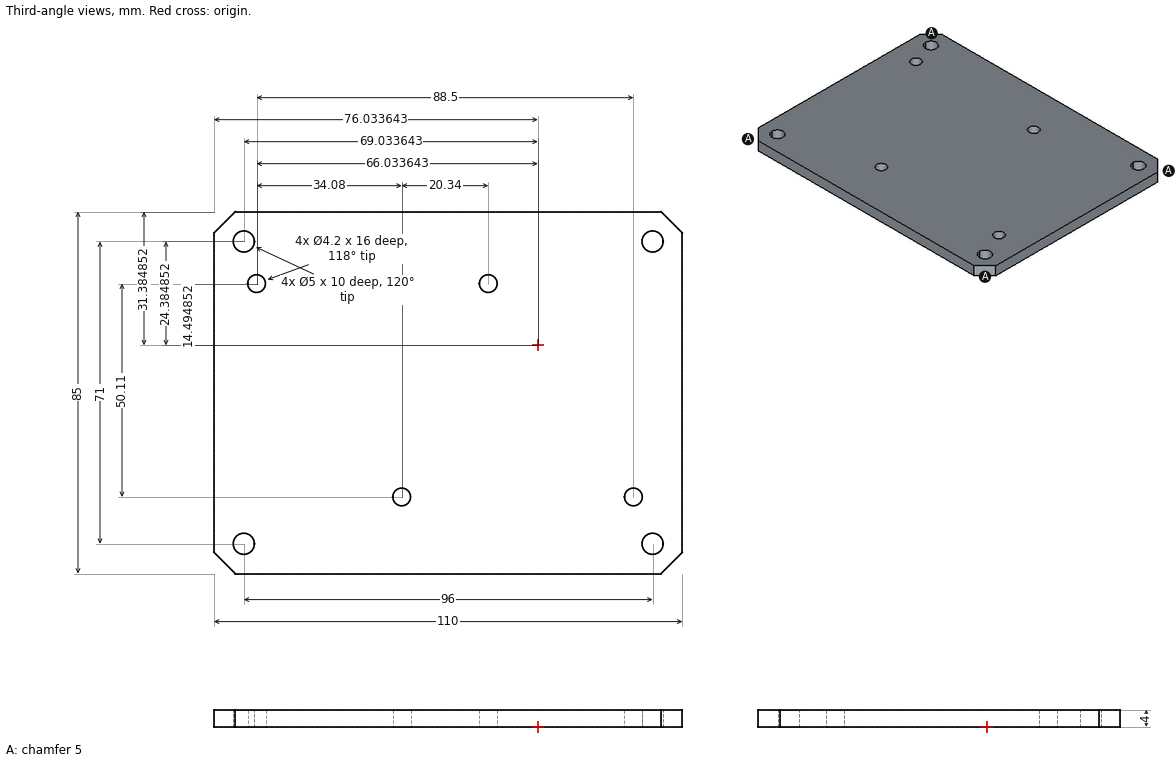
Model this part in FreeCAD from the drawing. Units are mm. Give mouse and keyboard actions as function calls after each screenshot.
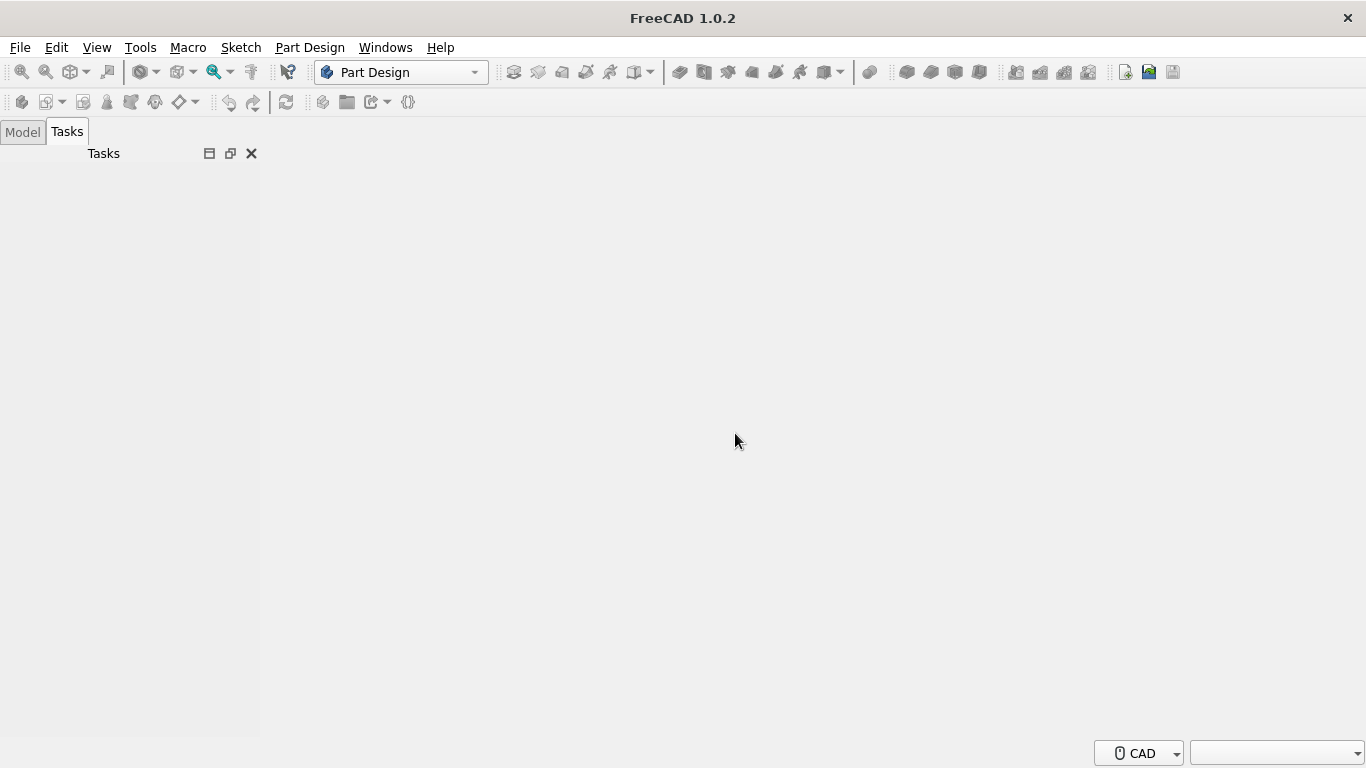
click(1126, 72)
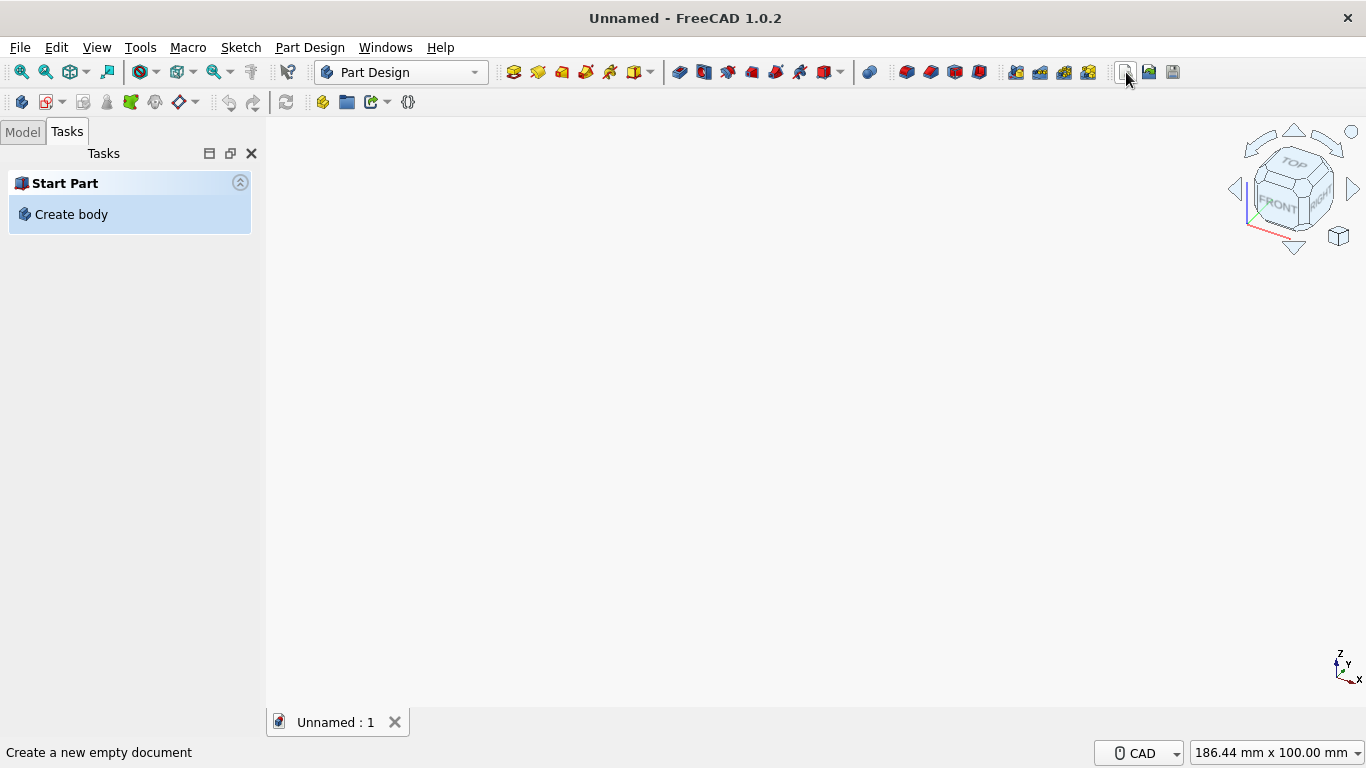
click(46, 102)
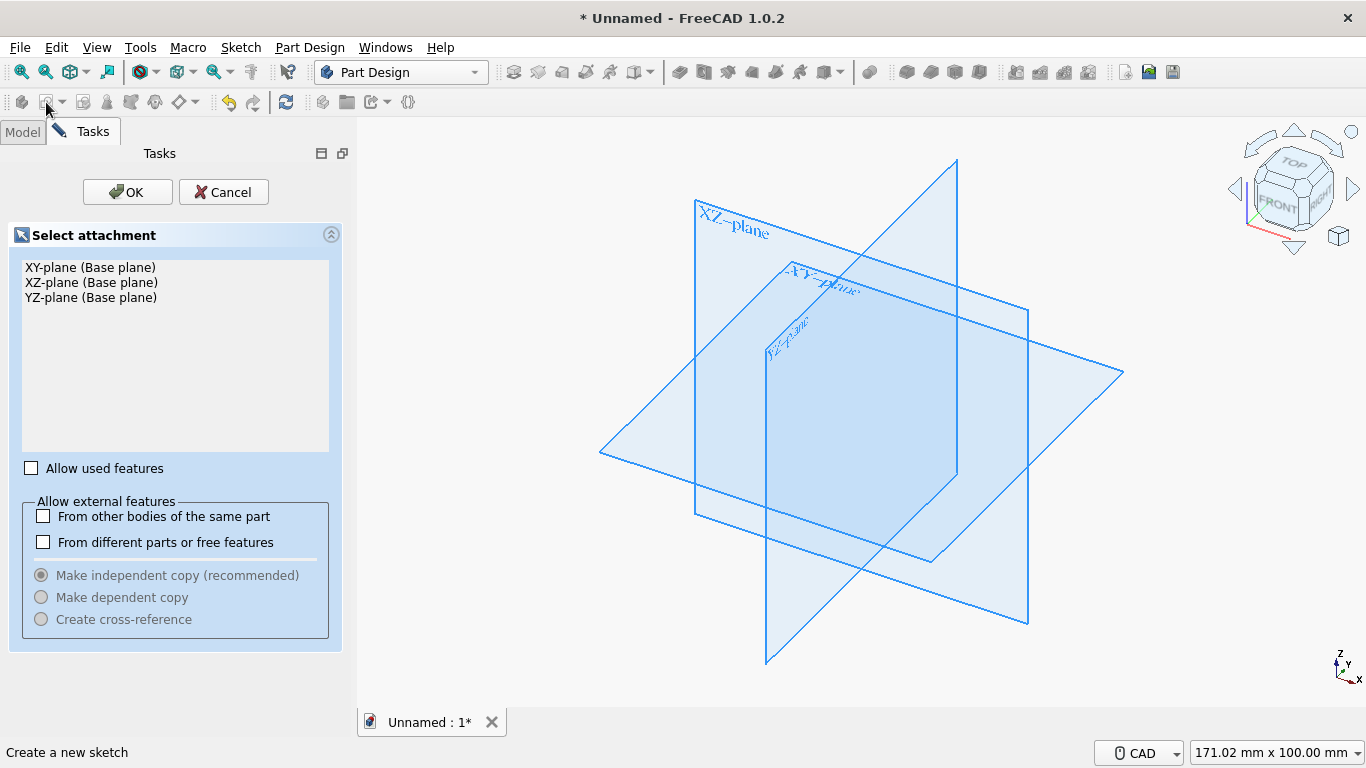
click(82, 268)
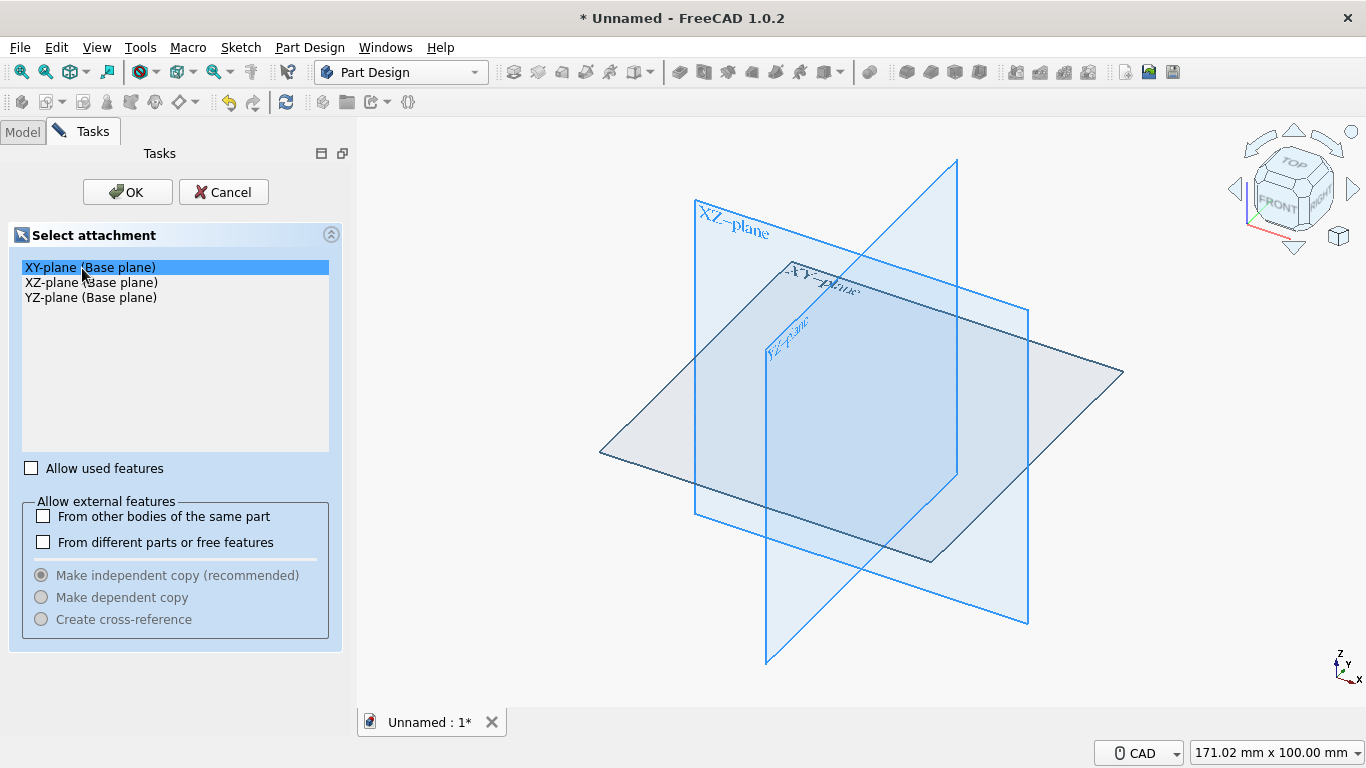
click(128, 192)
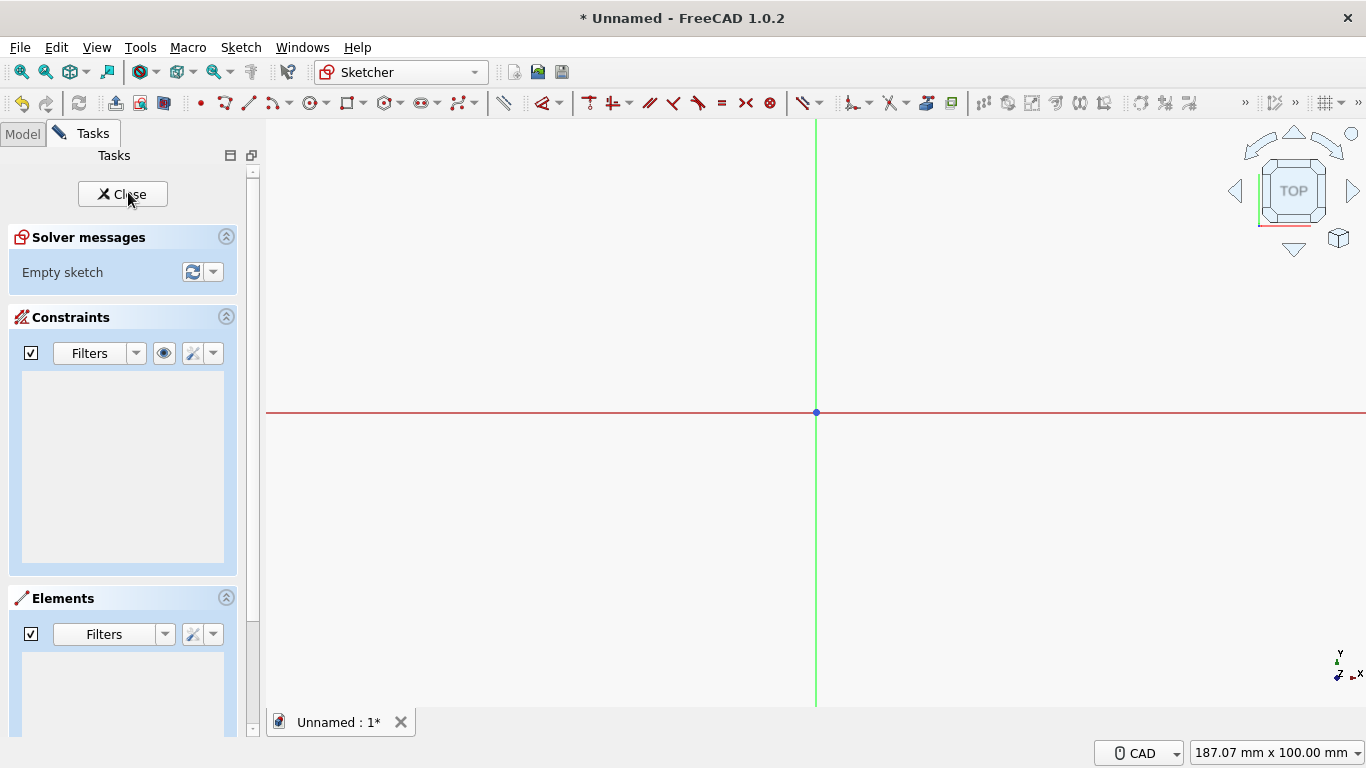
scroll(997, 147, down, 1)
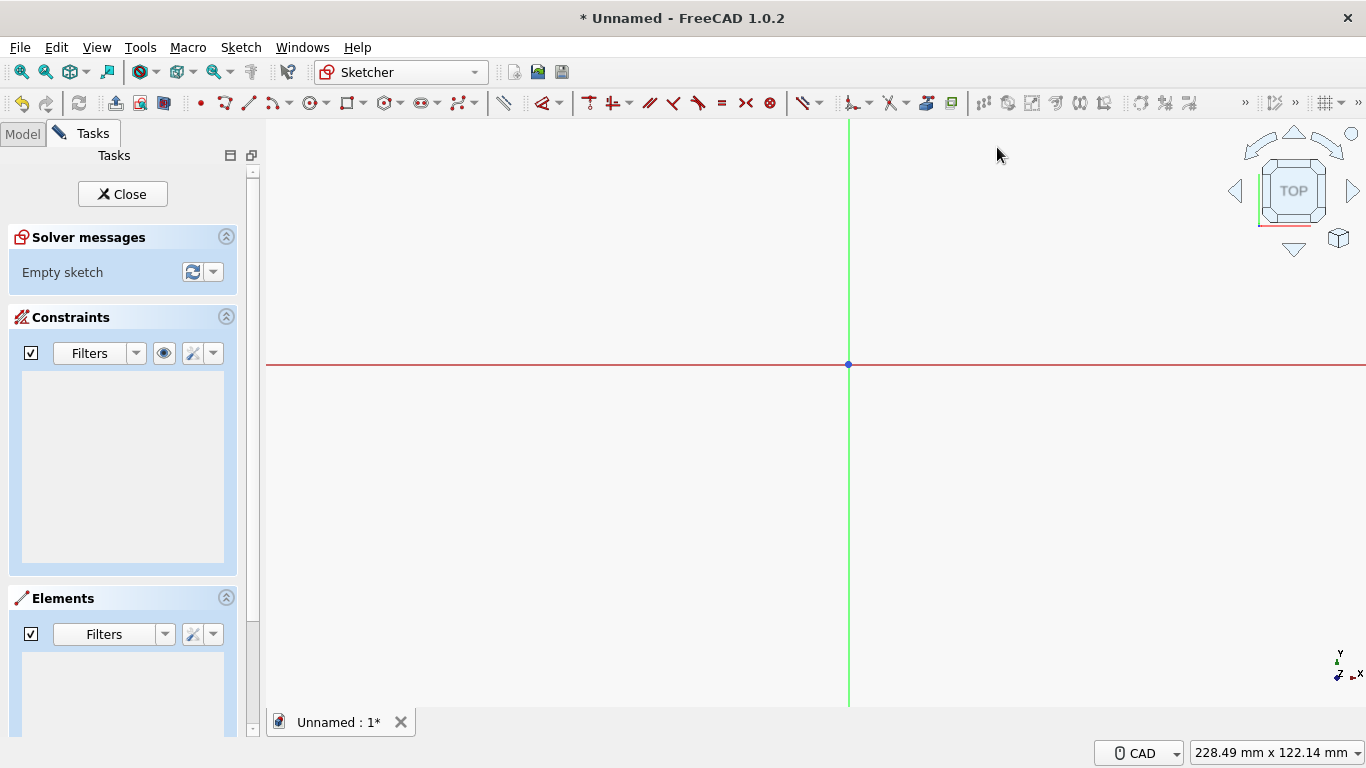
click(348, 104)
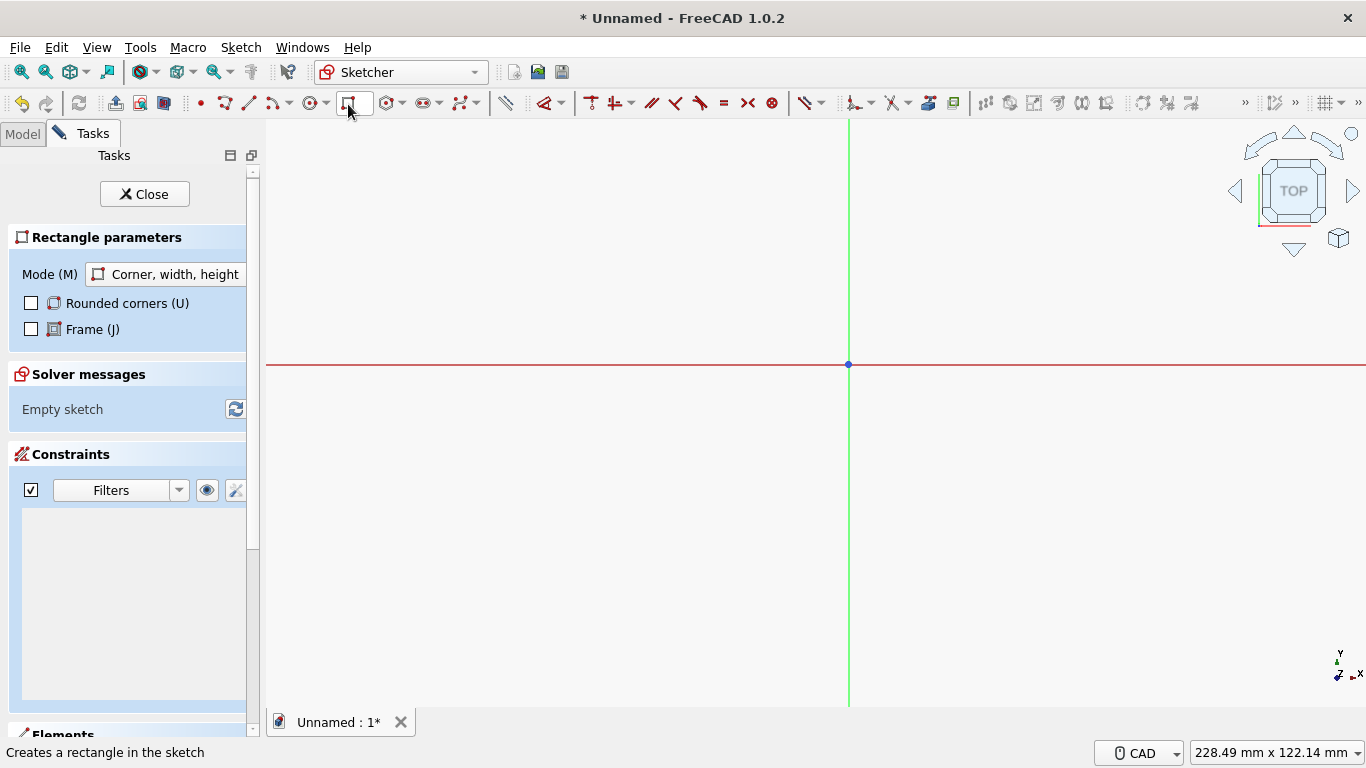
click(483, 214)
click(1012, 623)
key(Escape)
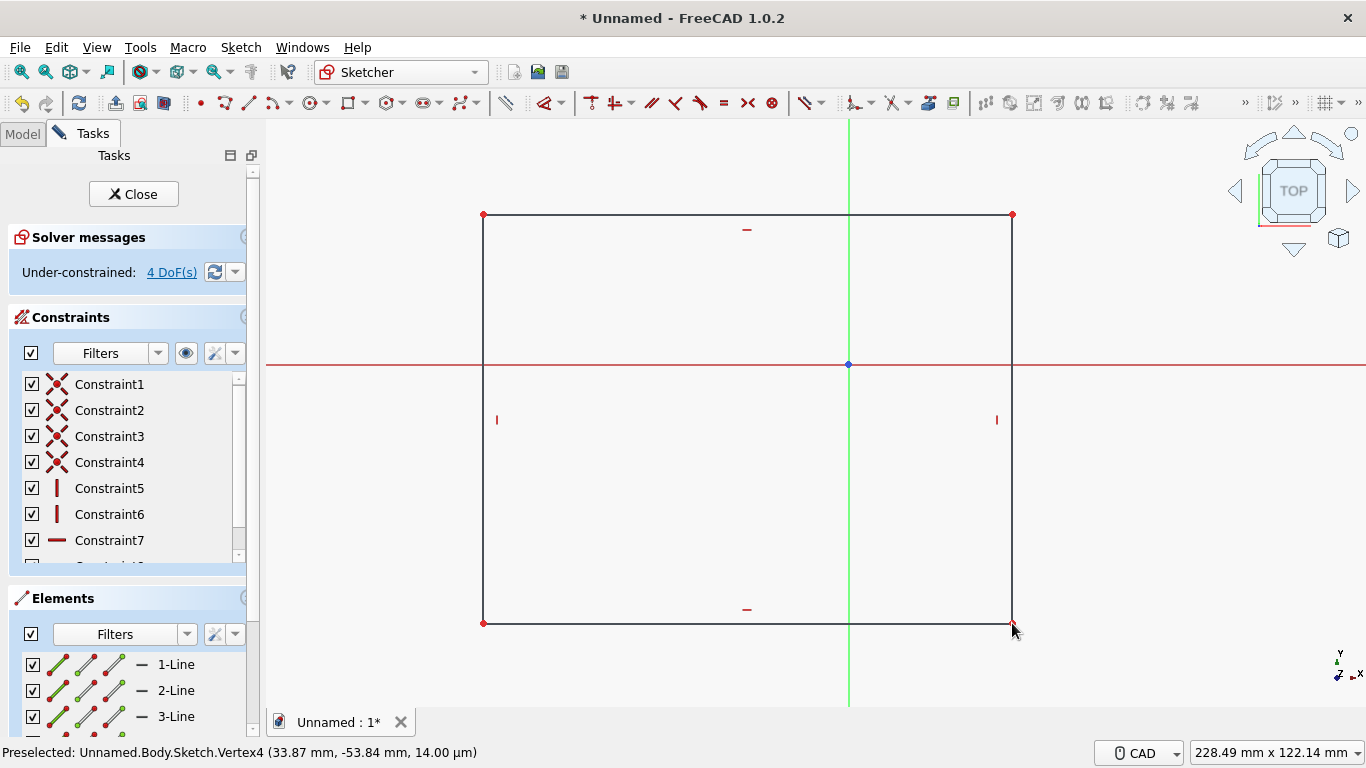
click(544, 104)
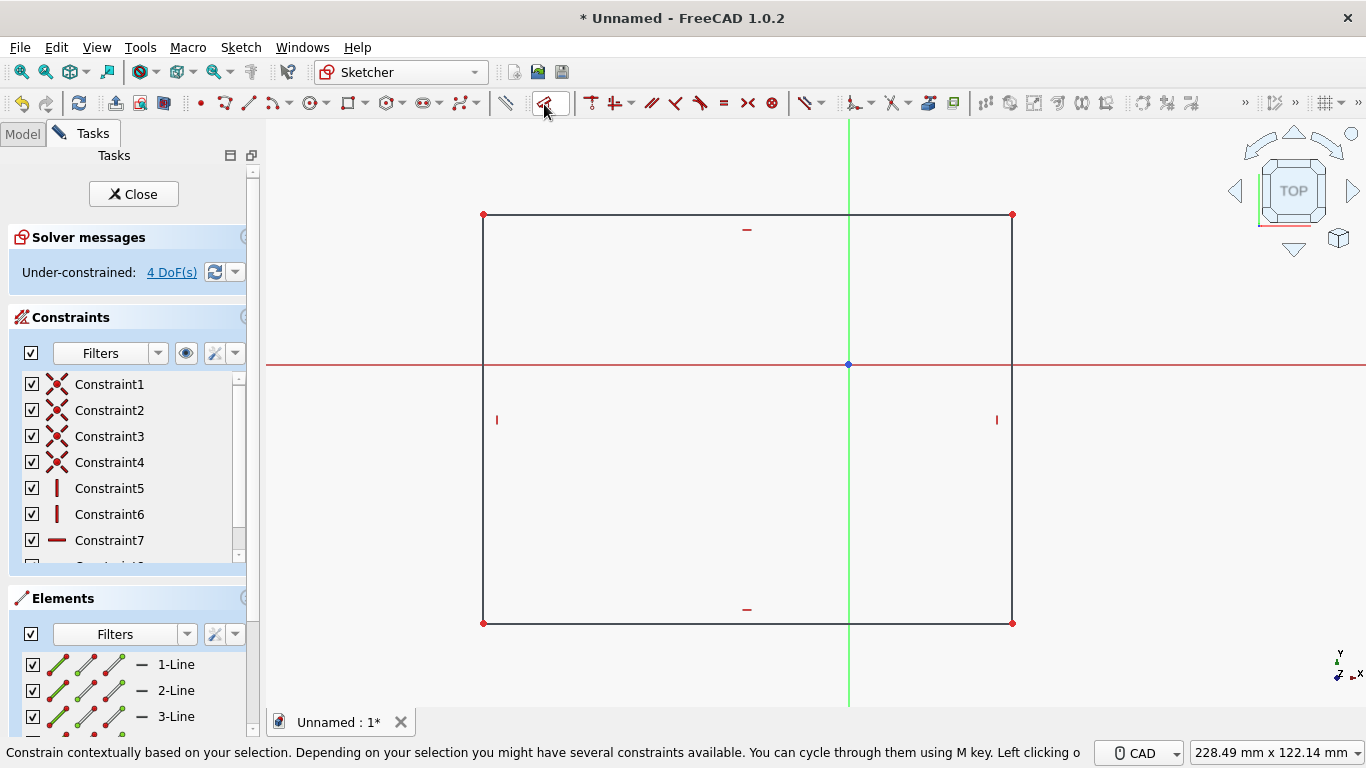
click(483, 338)
click(449, 419)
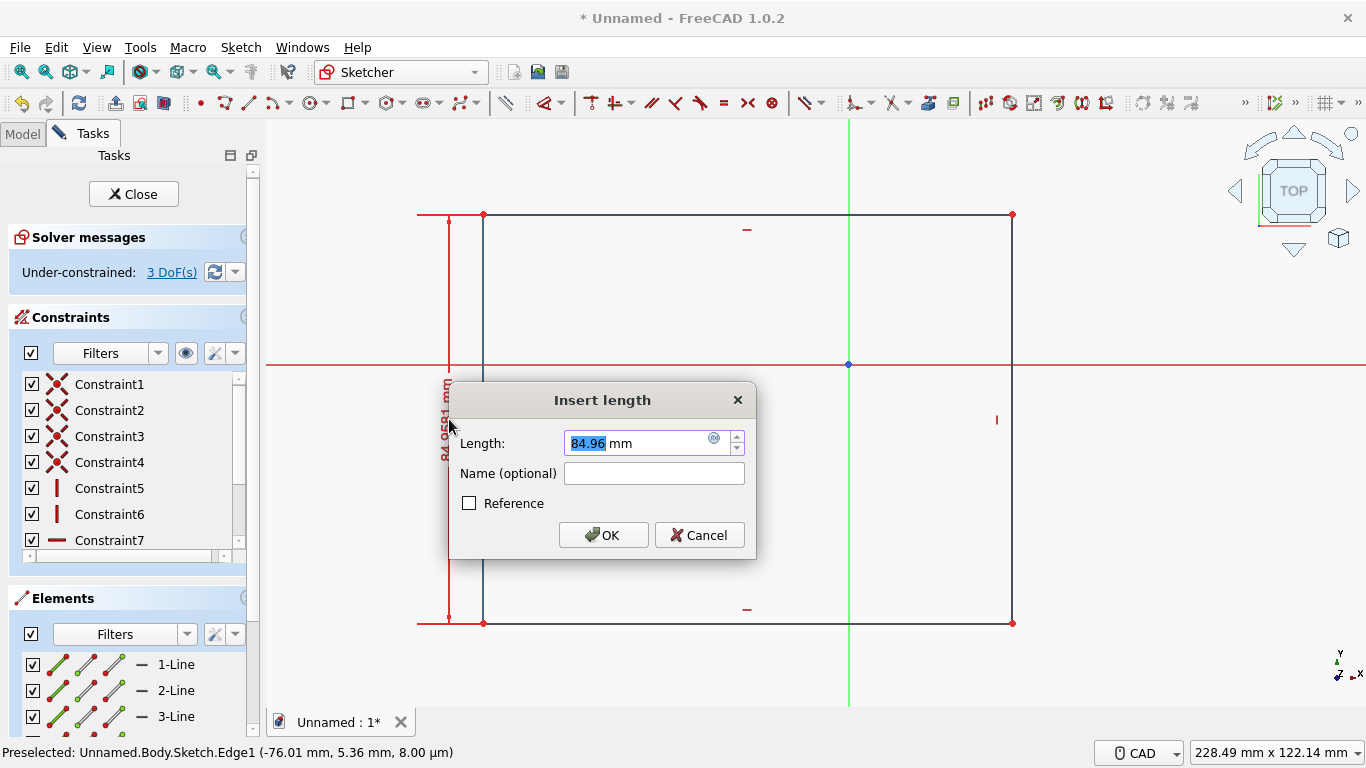
text(85)
key(Return)